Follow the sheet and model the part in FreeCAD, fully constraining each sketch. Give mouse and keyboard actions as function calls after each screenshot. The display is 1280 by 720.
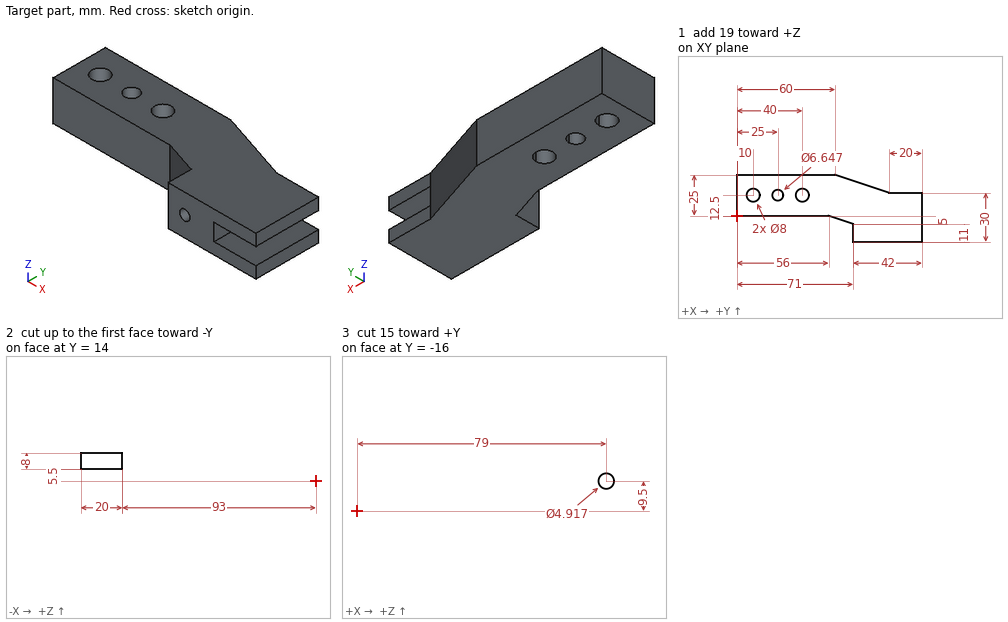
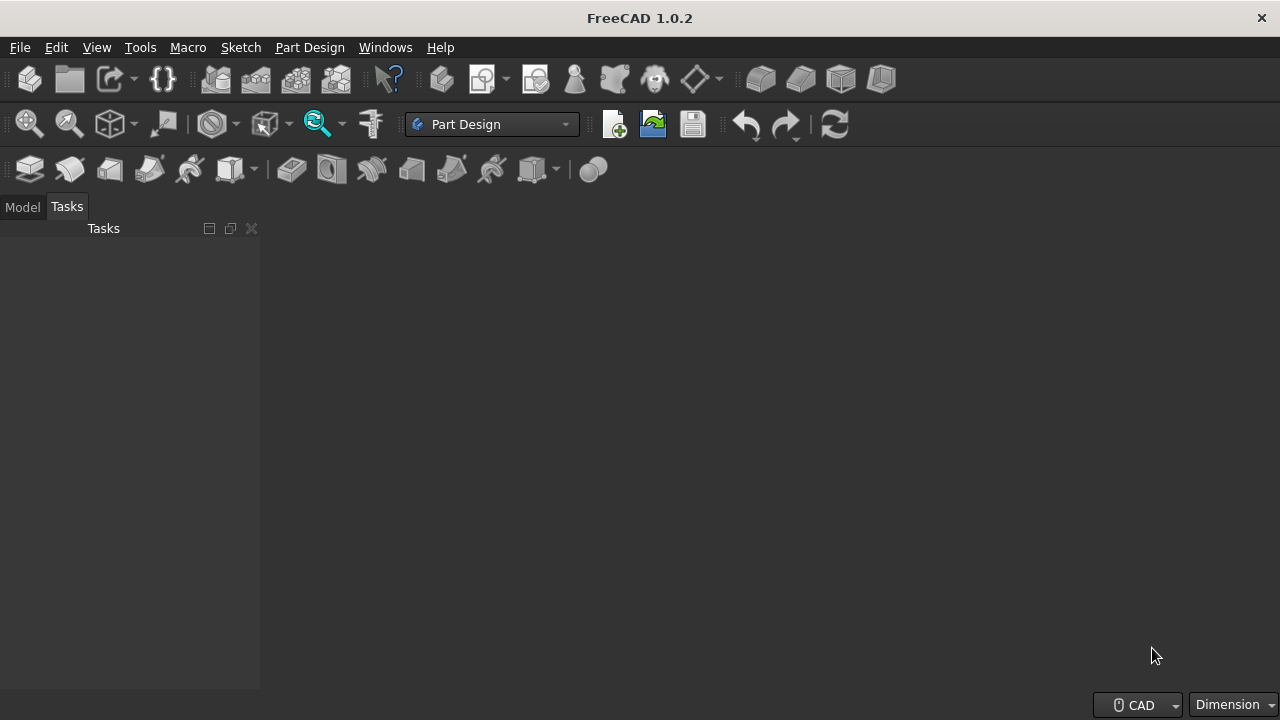
click(614, 124)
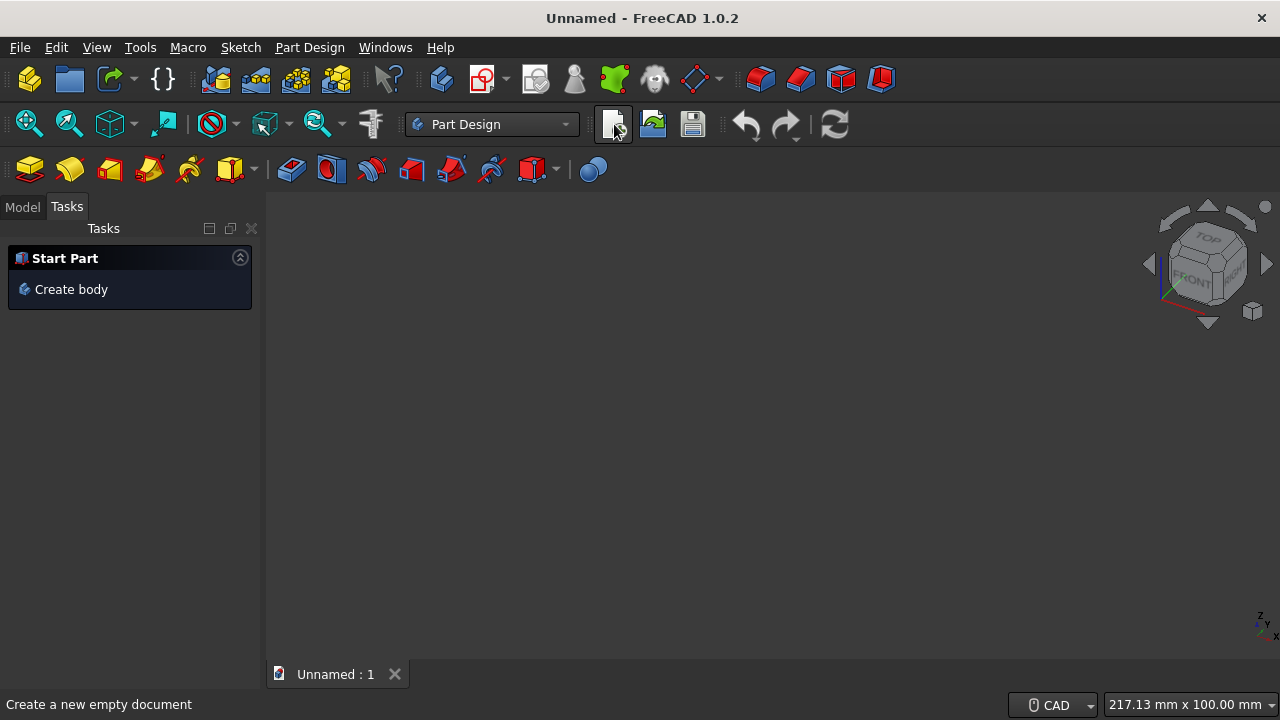
click(482, 80)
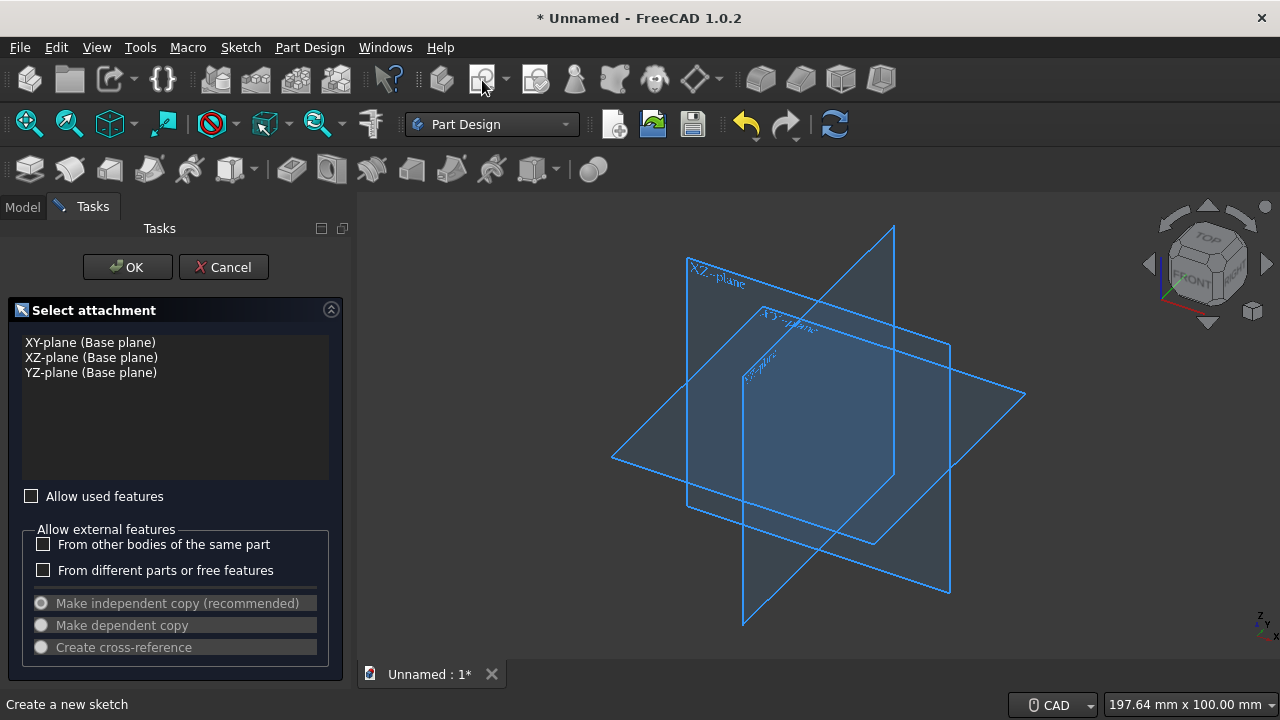
click(82, 342)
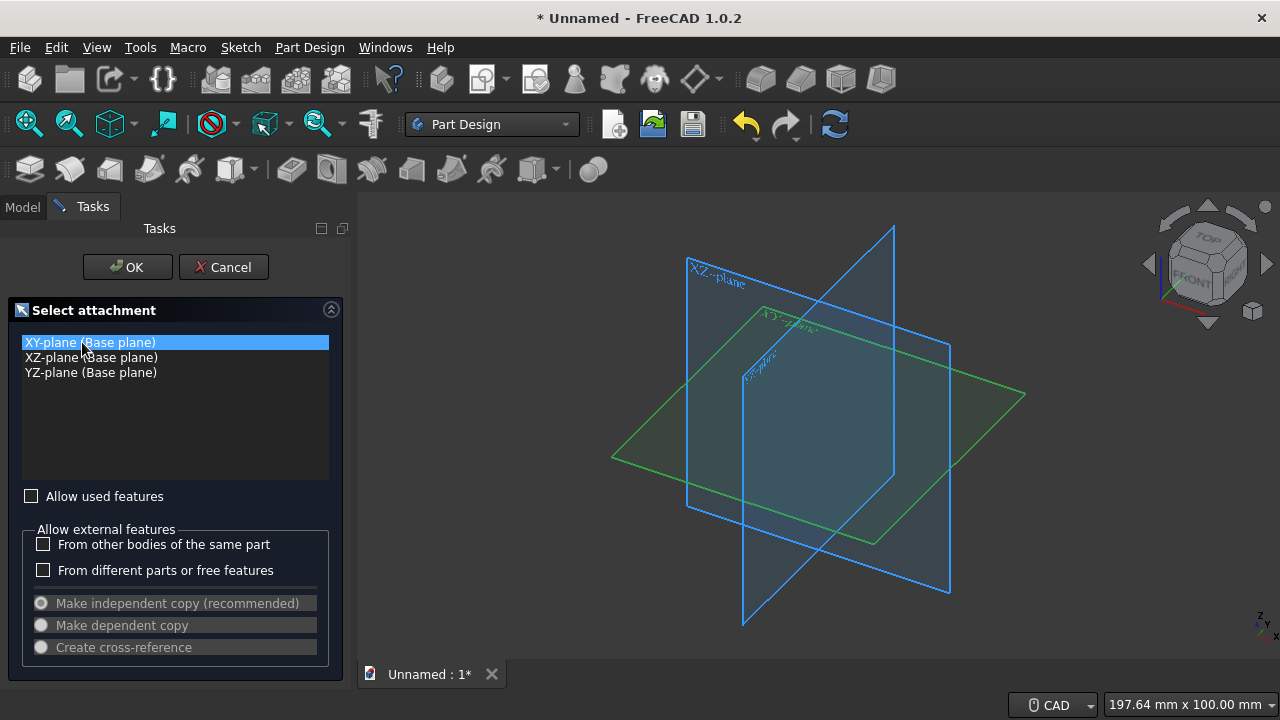
click(128, 267)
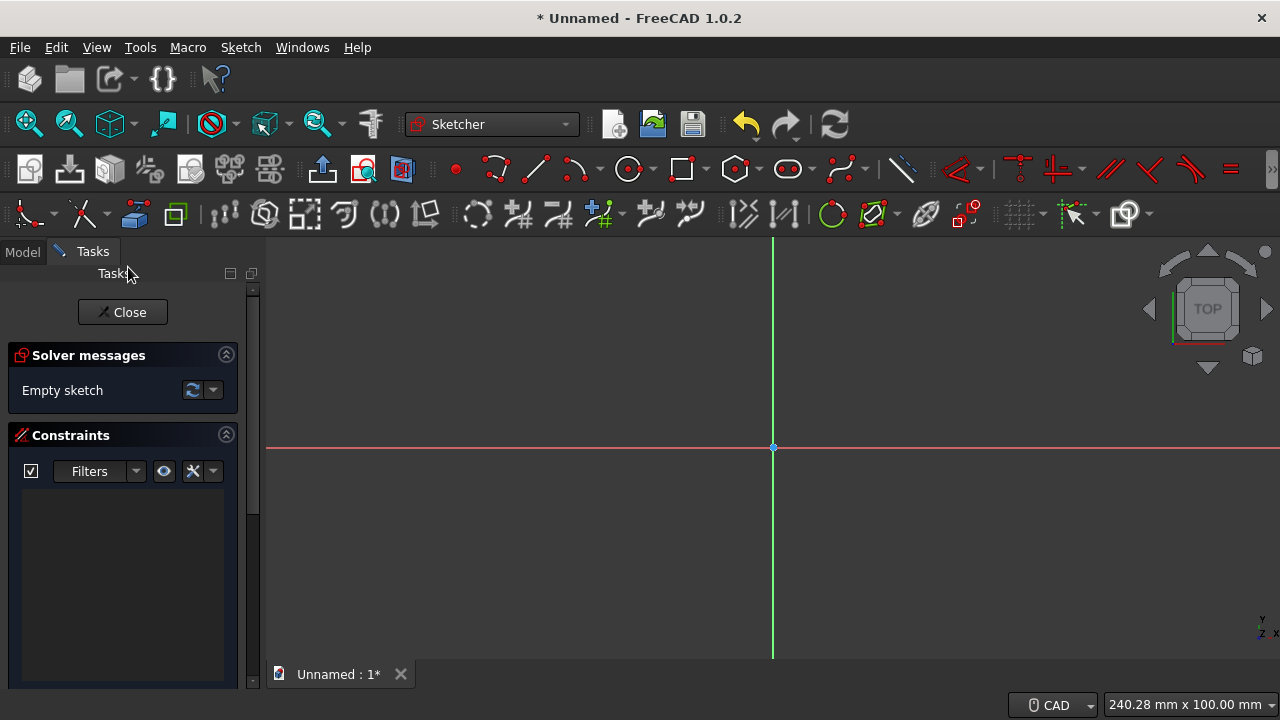
scroll(294, 534, down, 1)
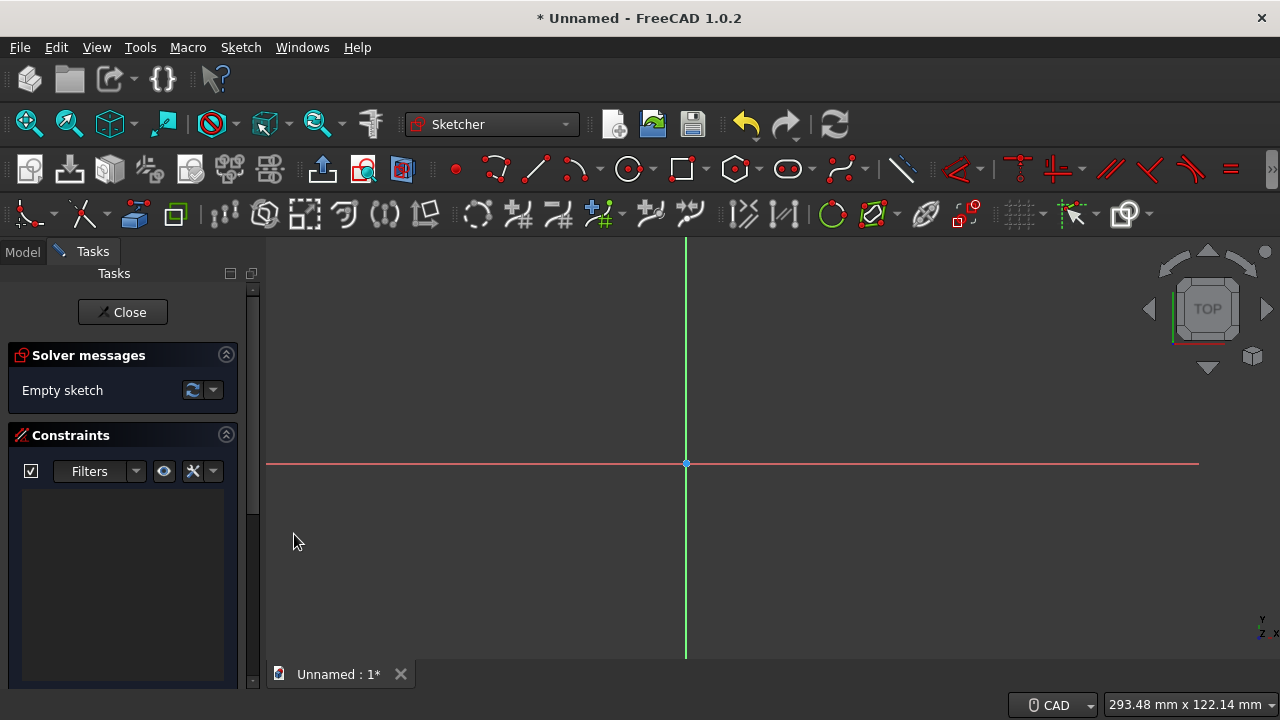
scroll(1115, 449, up, 2)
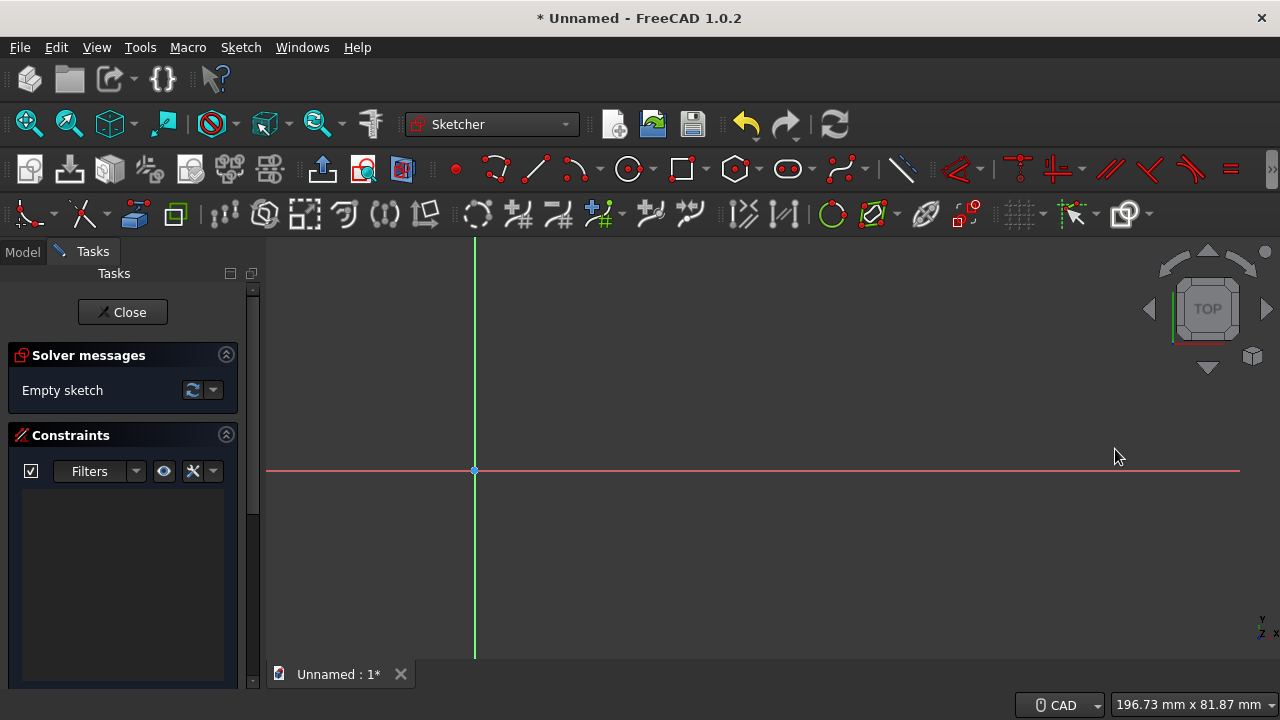
click(496, 170)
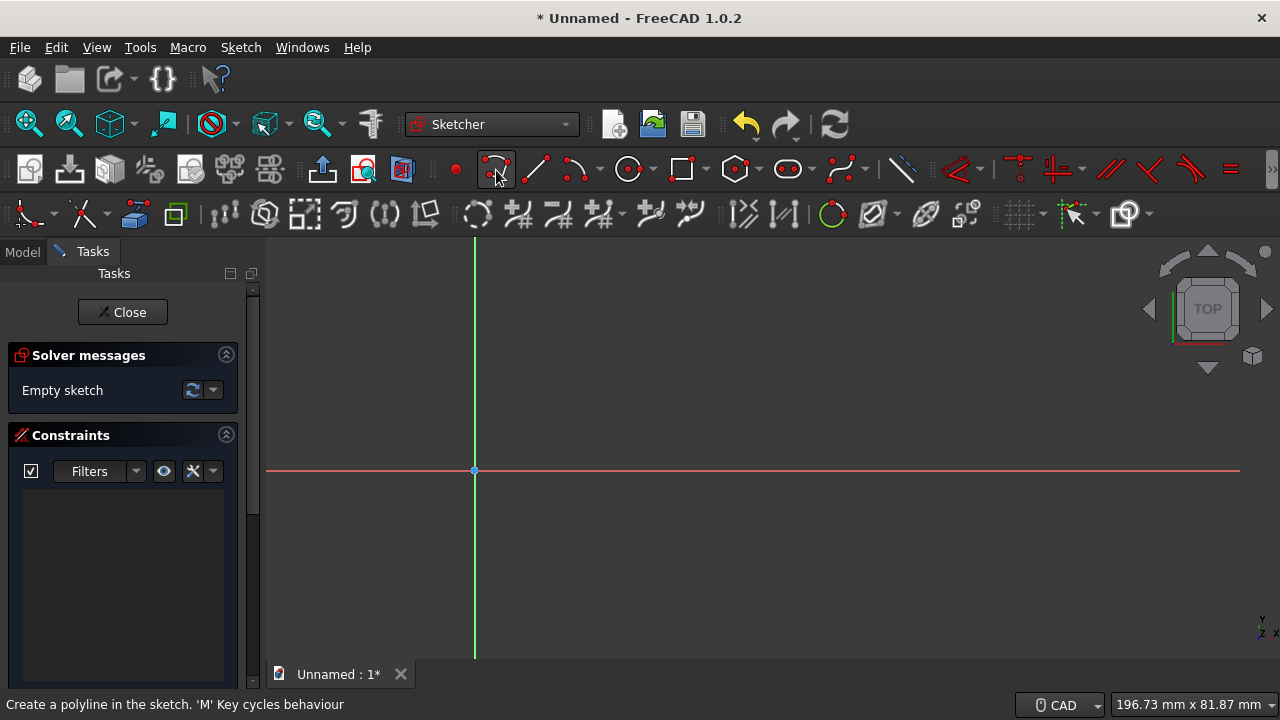
click(475, 471)
click(764, 462)
click(841, 496)
click(841, 553)
click(1057, 553)
click(1057, 399)
click(954, 399)
click(784, 342)
click(484, 342)
click(475, 471)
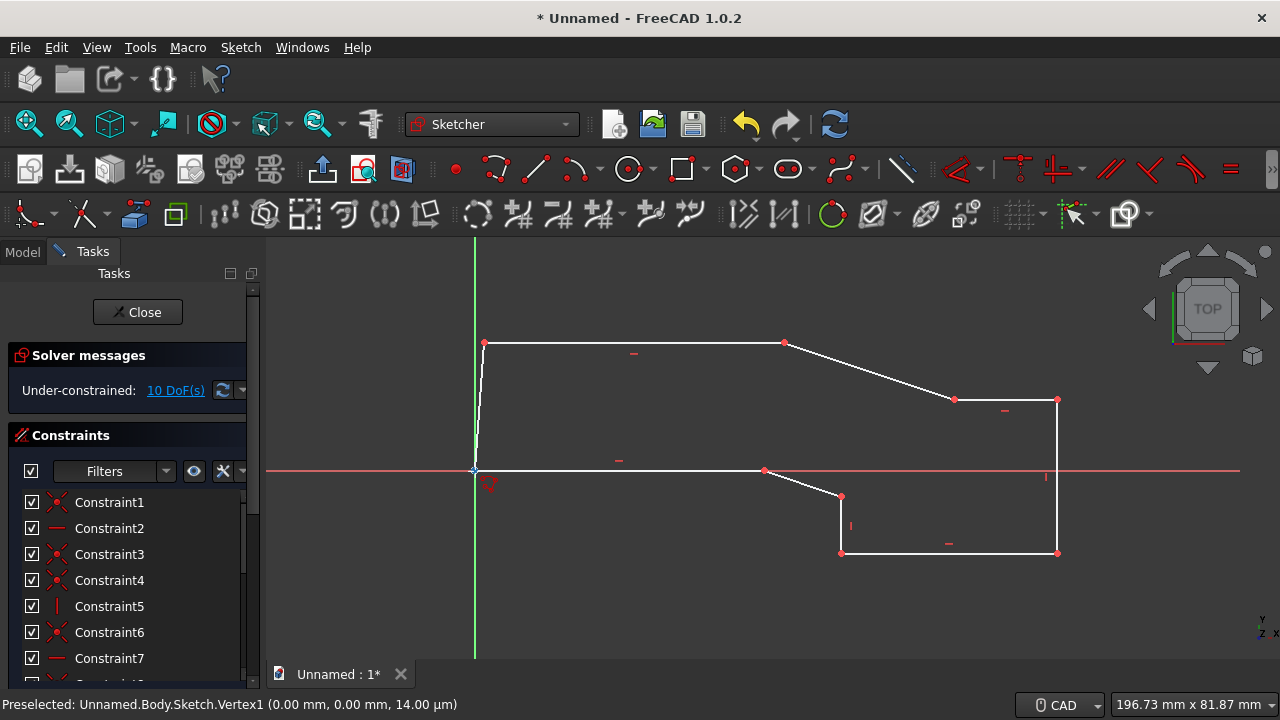
key(g)
key(c)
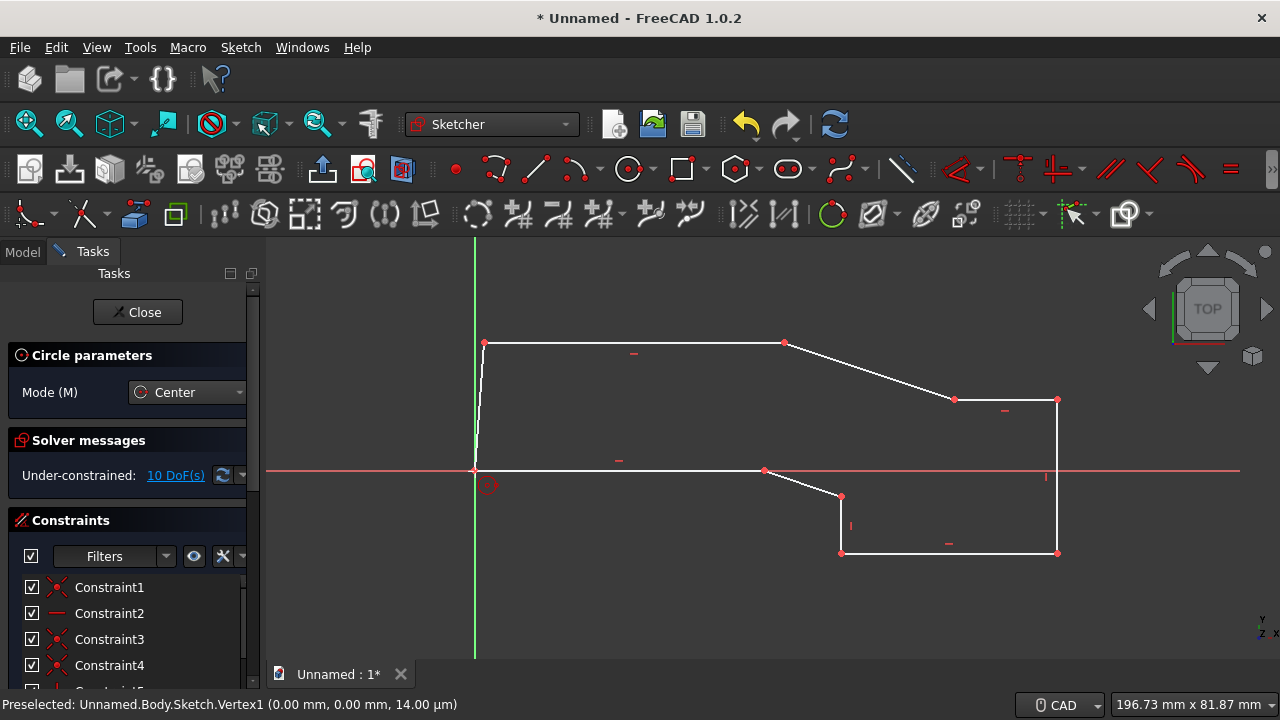
click(526, 406)
click(541, 392)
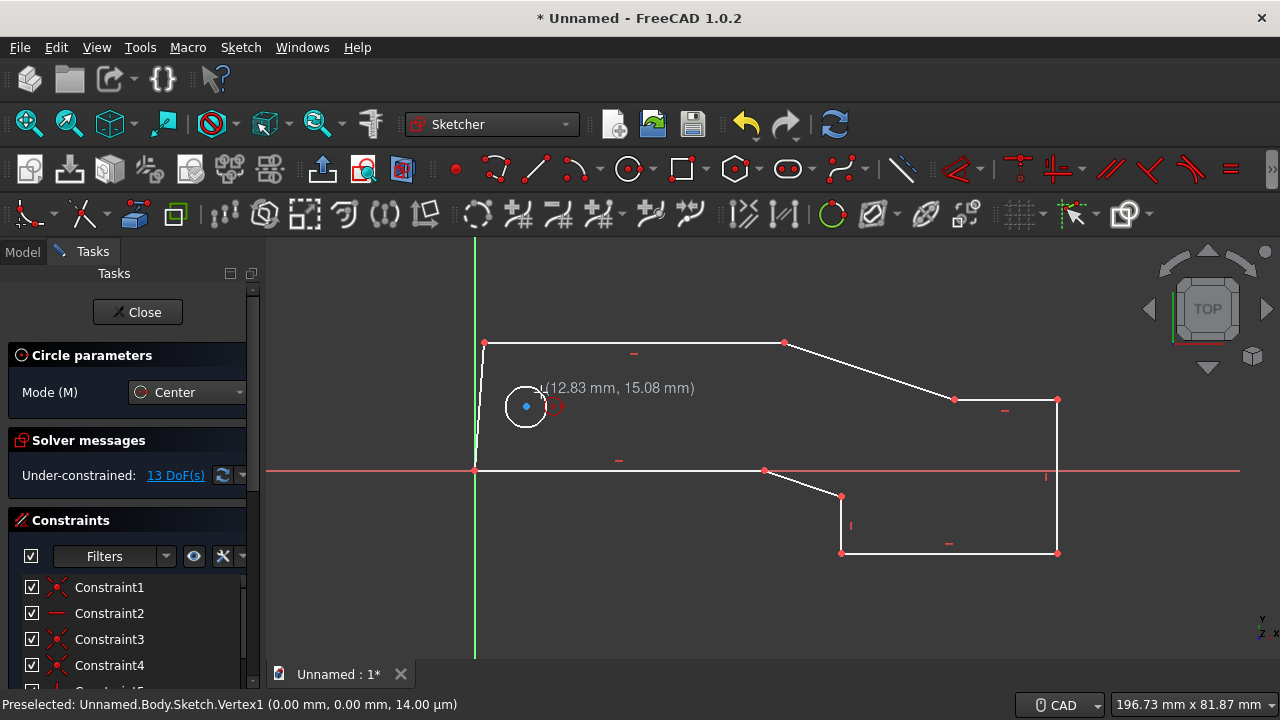
scroll(604, 406, up, 2)